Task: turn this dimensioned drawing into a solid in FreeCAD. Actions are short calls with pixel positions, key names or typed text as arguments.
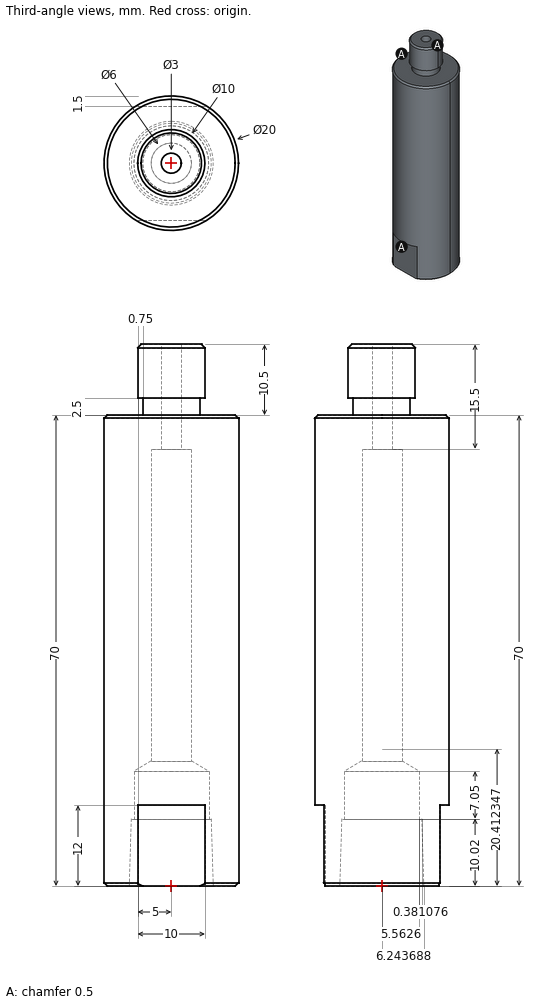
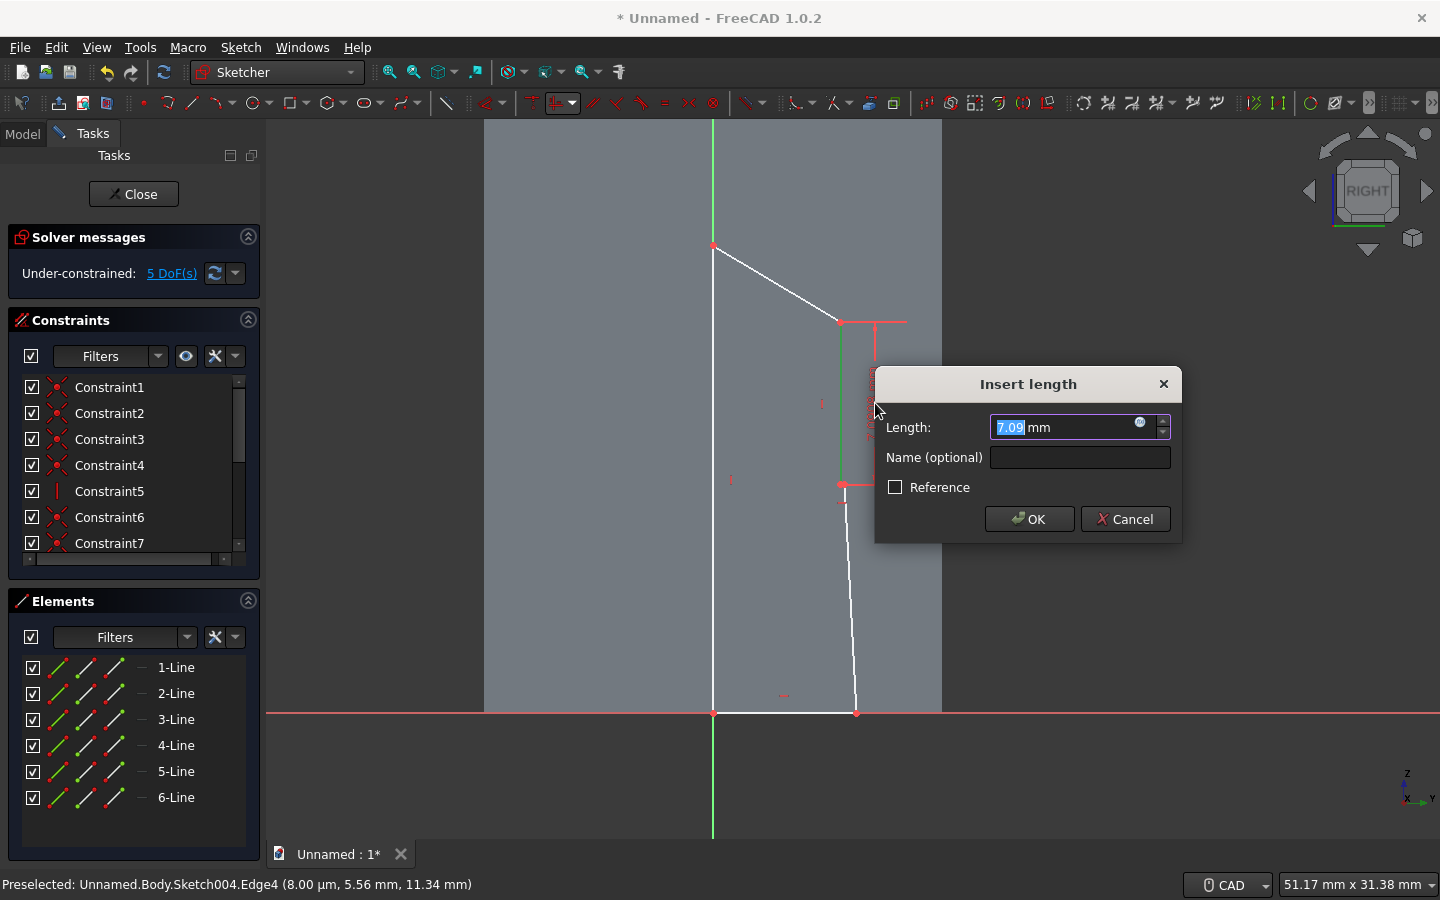
text(7.05)
key(Return)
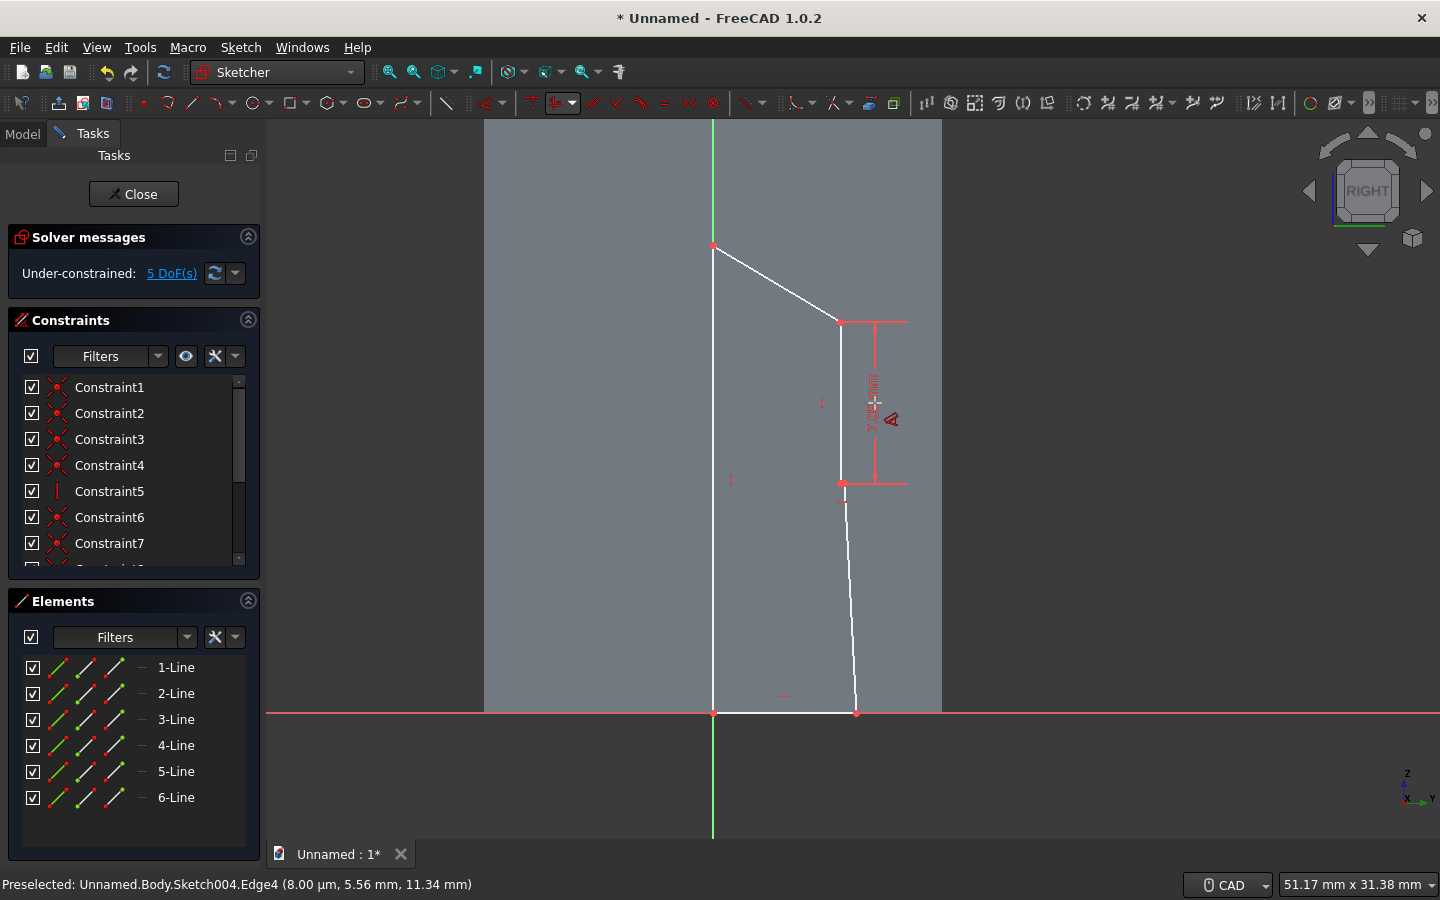
scroll(845, 484, up, 6)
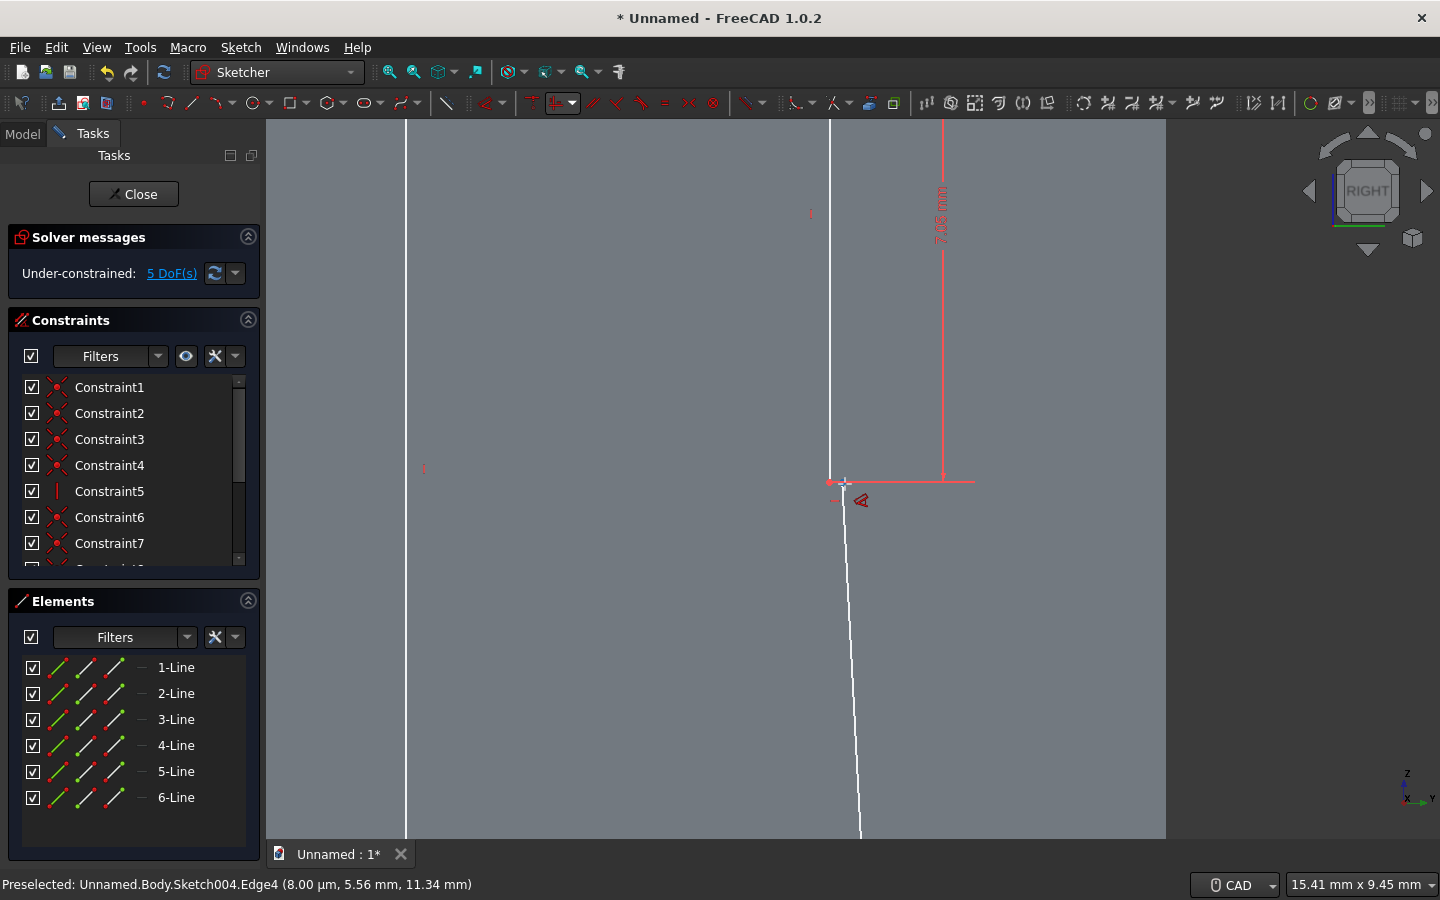
click(842, 482)
click(372, 647)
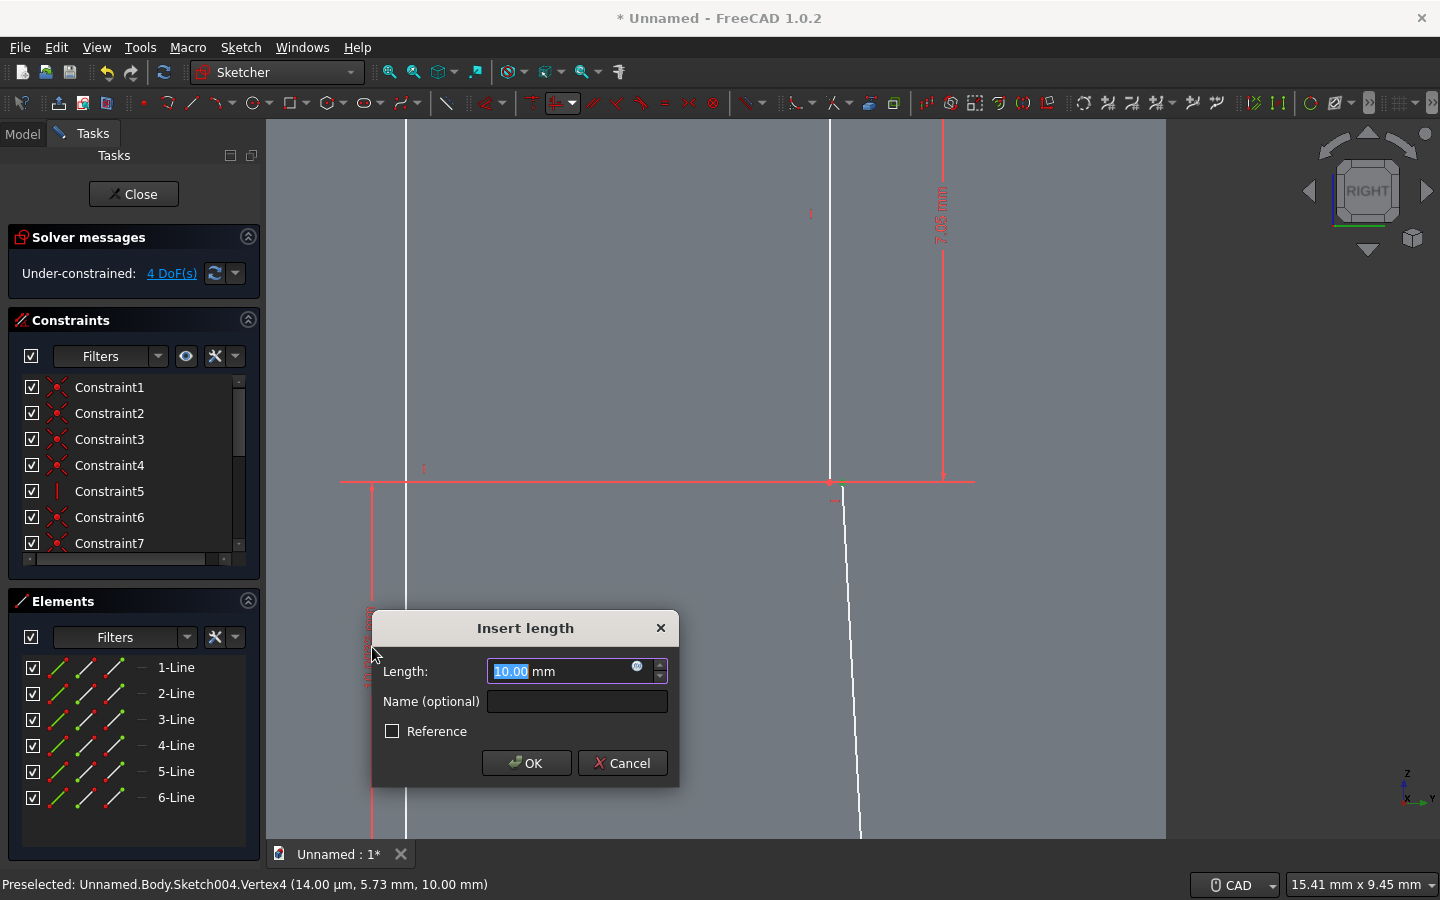
text(10.02)
key(Return)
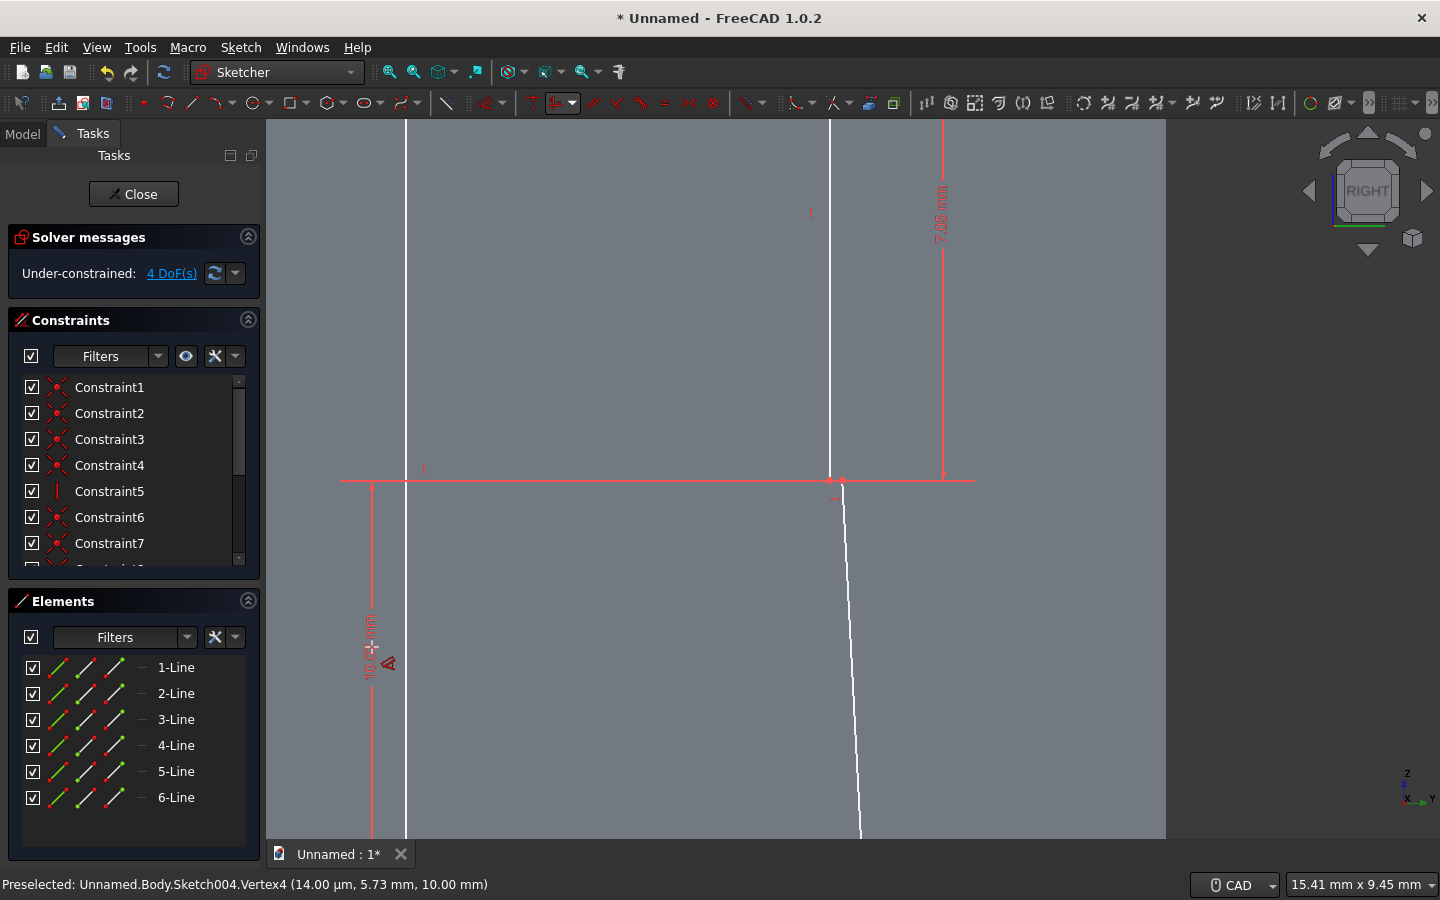
click(830, 481)
click(618, 447)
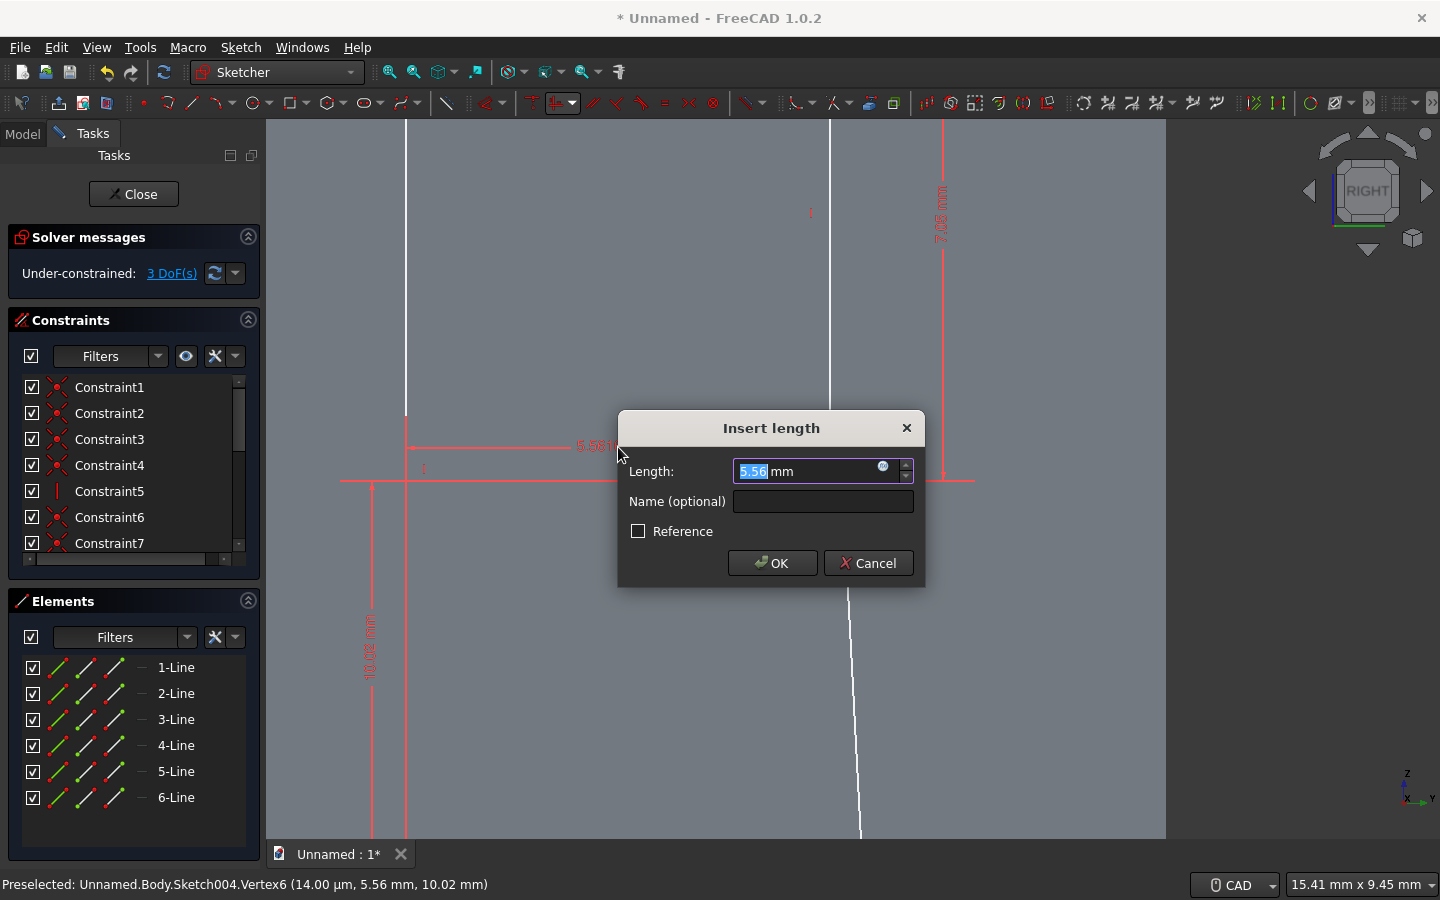
text(5.5626)
key(Return)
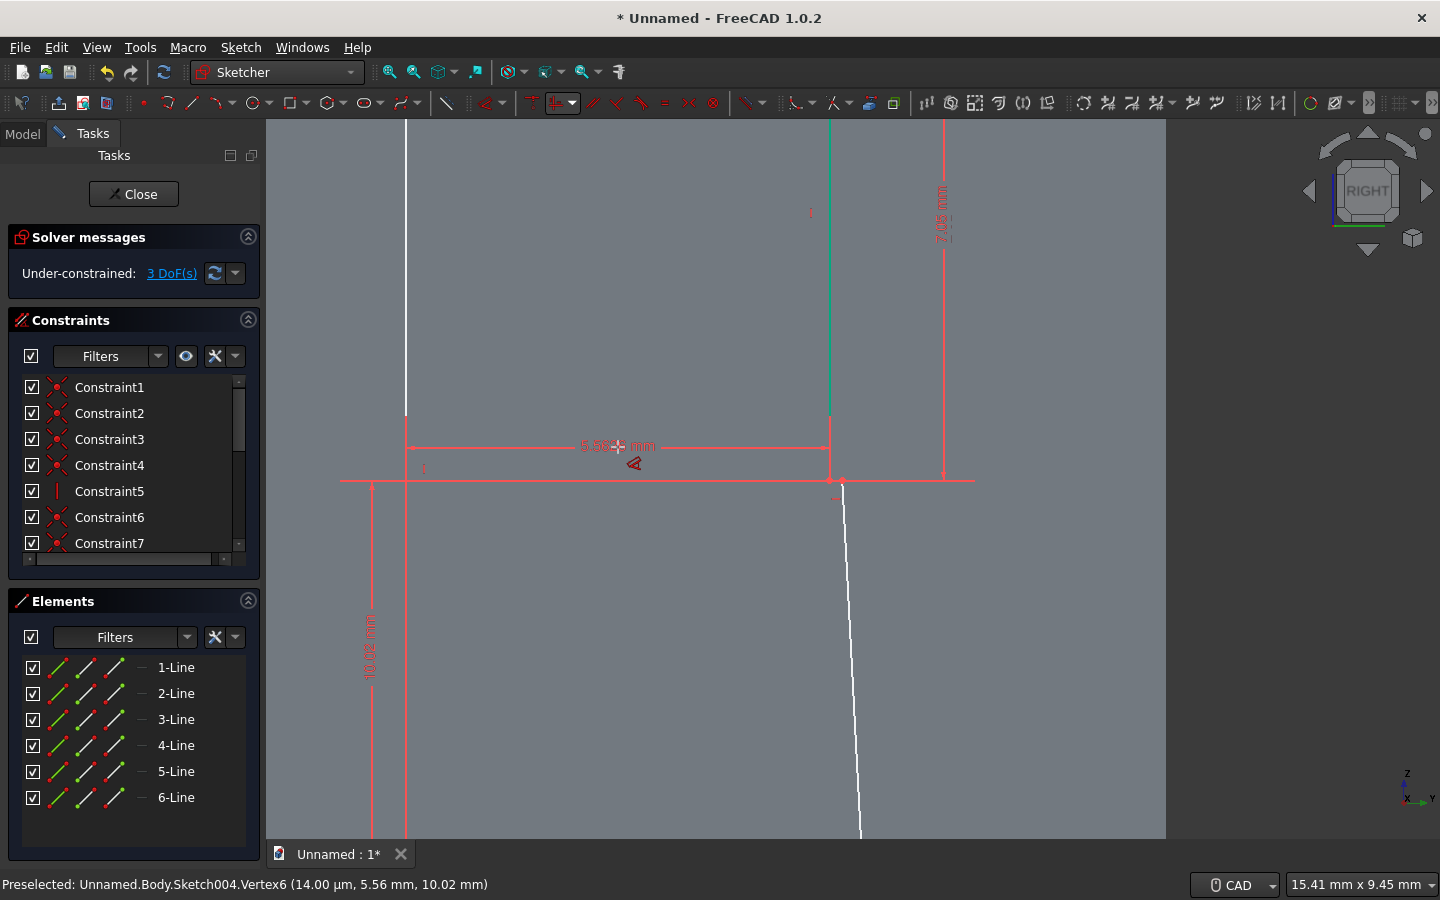
scroll(845, 484, down, 6)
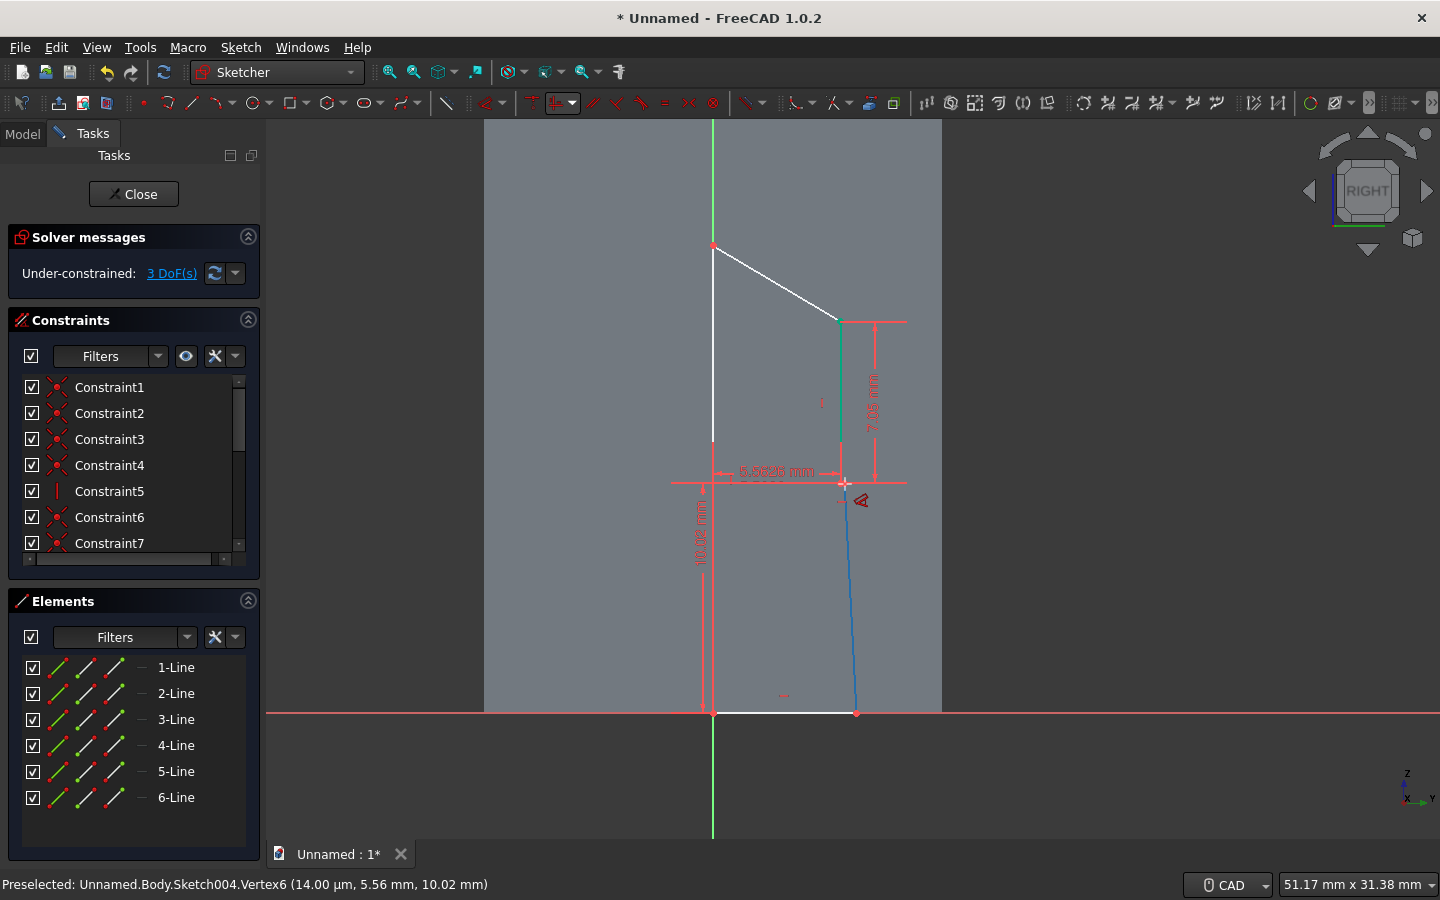
click(756, 713)
click(785, 747)